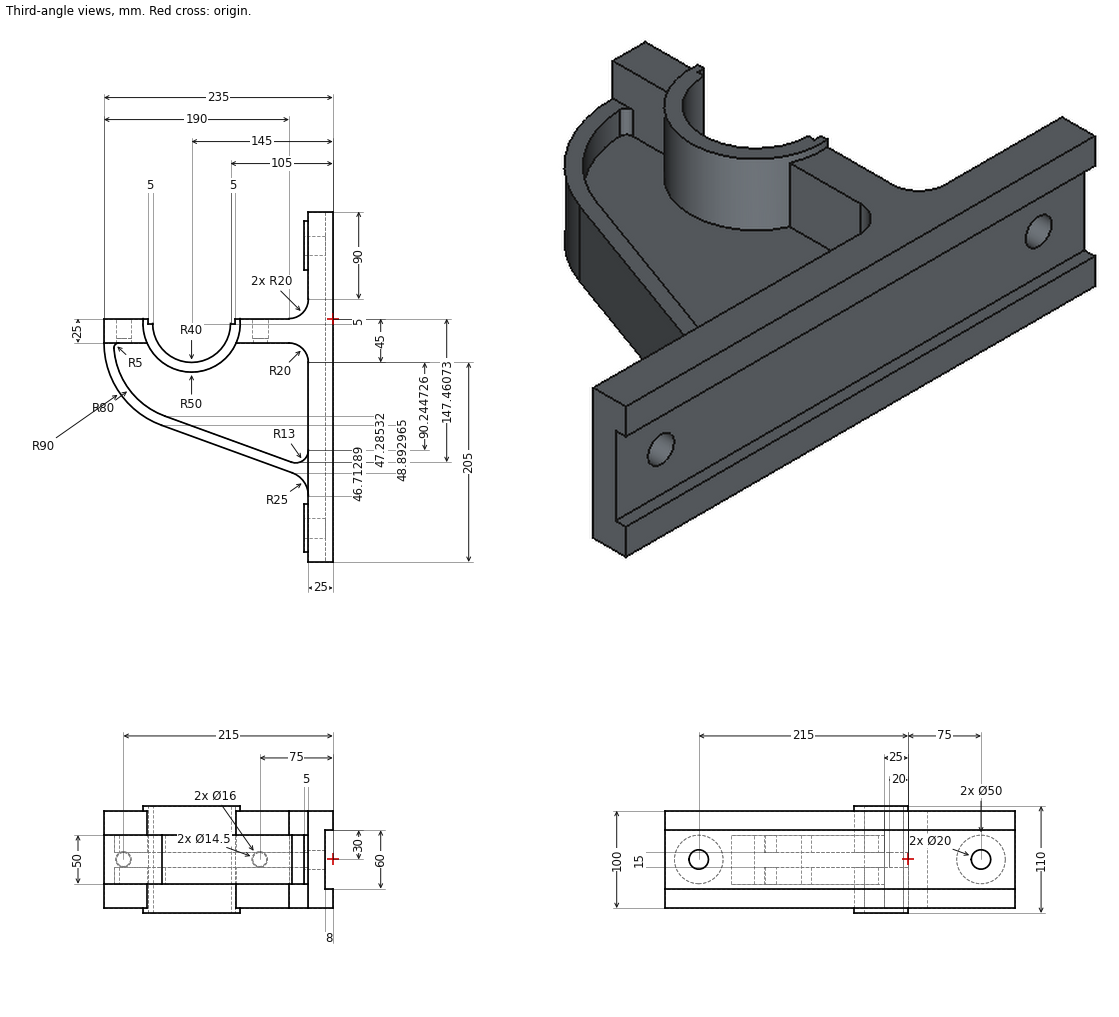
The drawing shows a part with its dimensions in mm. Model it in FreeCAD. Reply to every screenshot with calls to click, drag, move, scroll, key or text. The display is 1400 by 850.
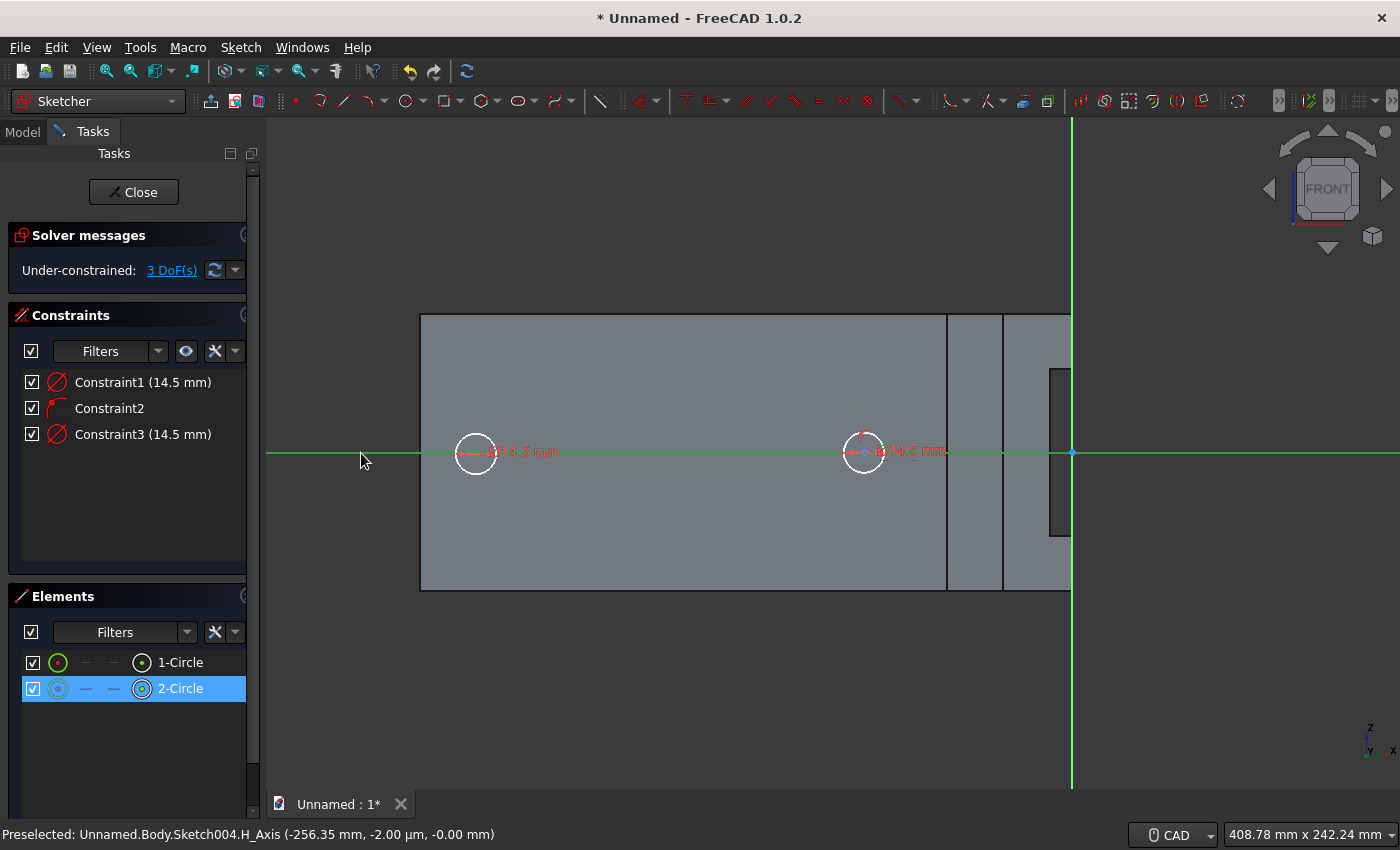
click(686, 102)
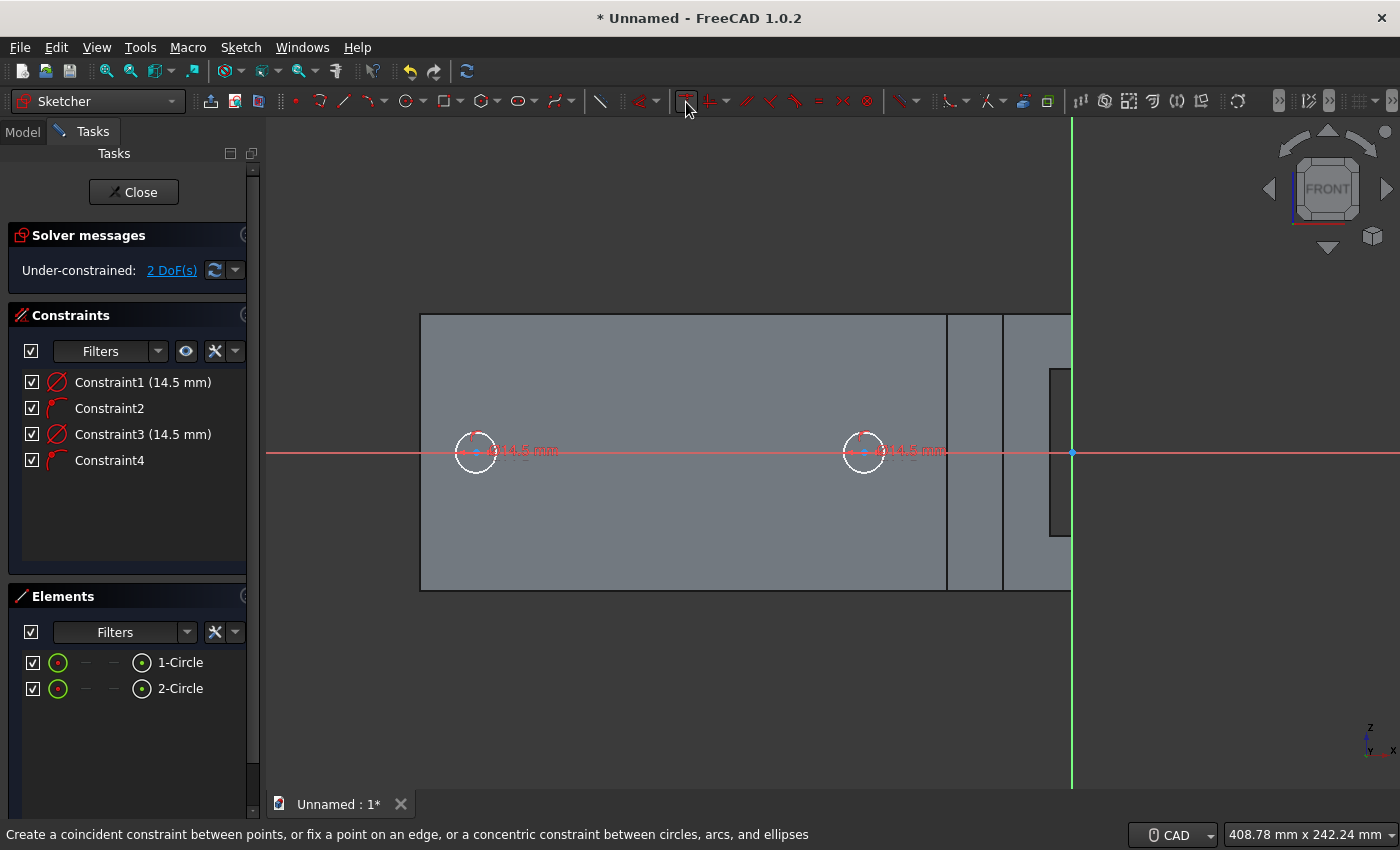
click(640, 102)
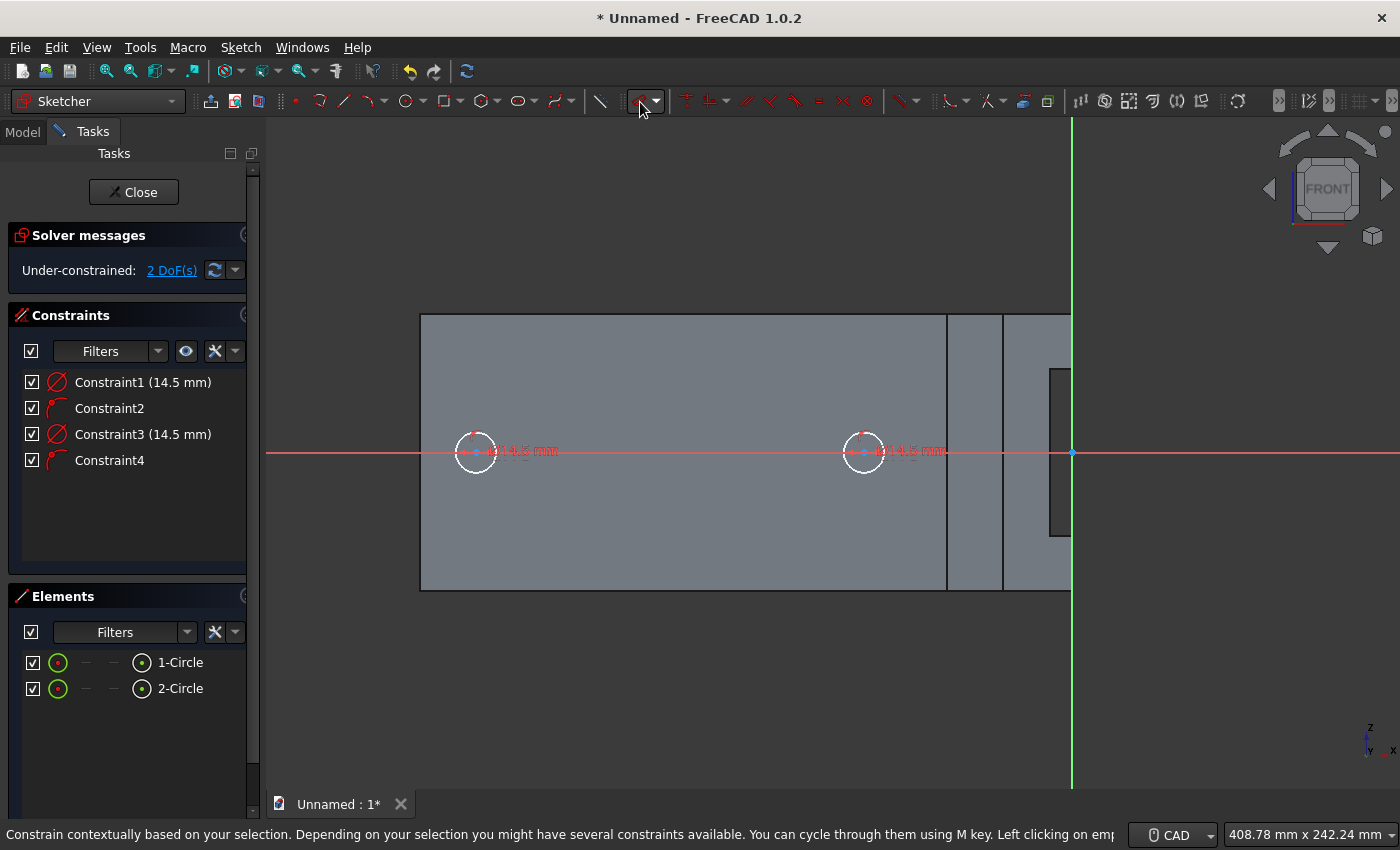
click(864, 453)
click(968, 487)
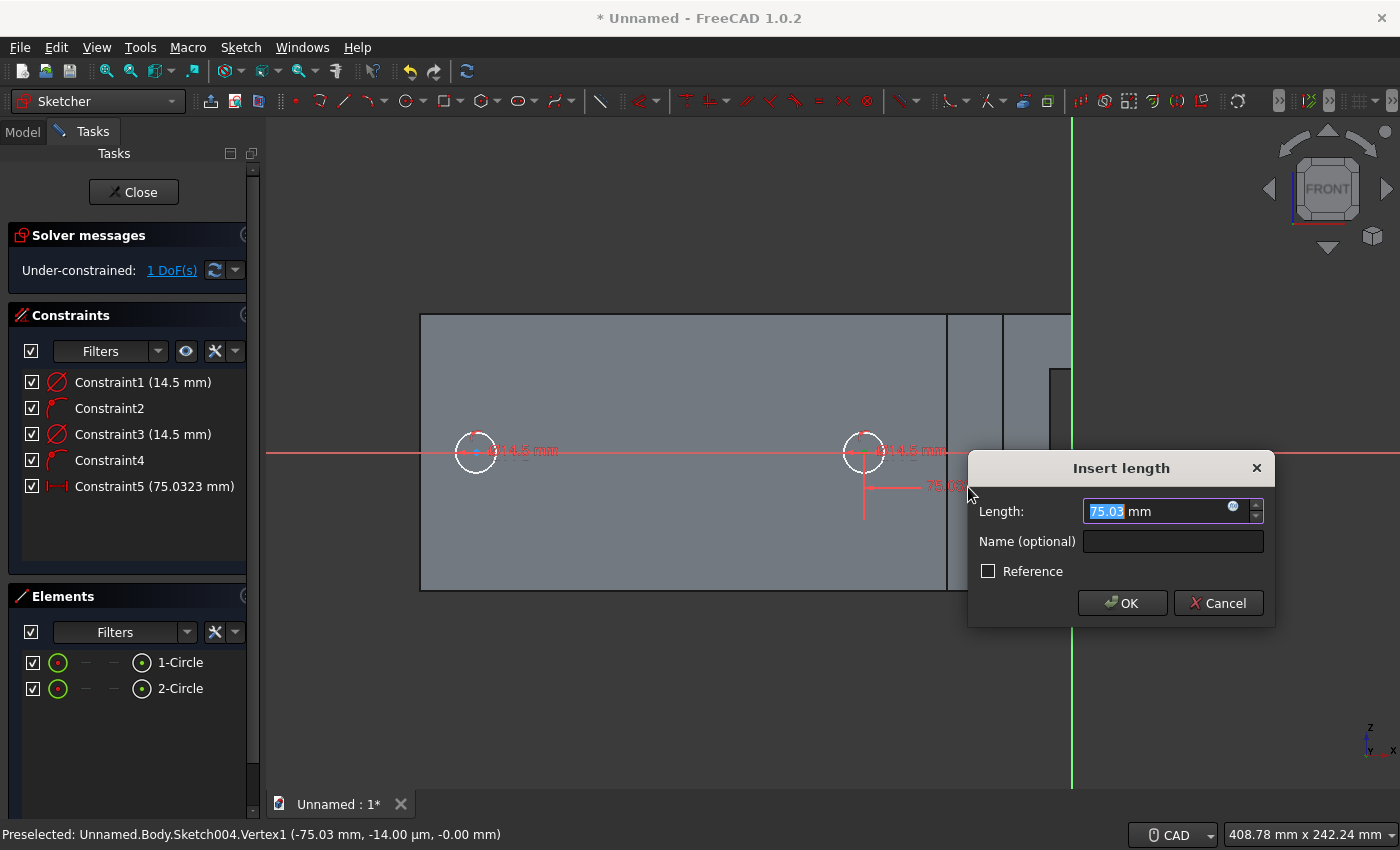
text(75)
key(Return)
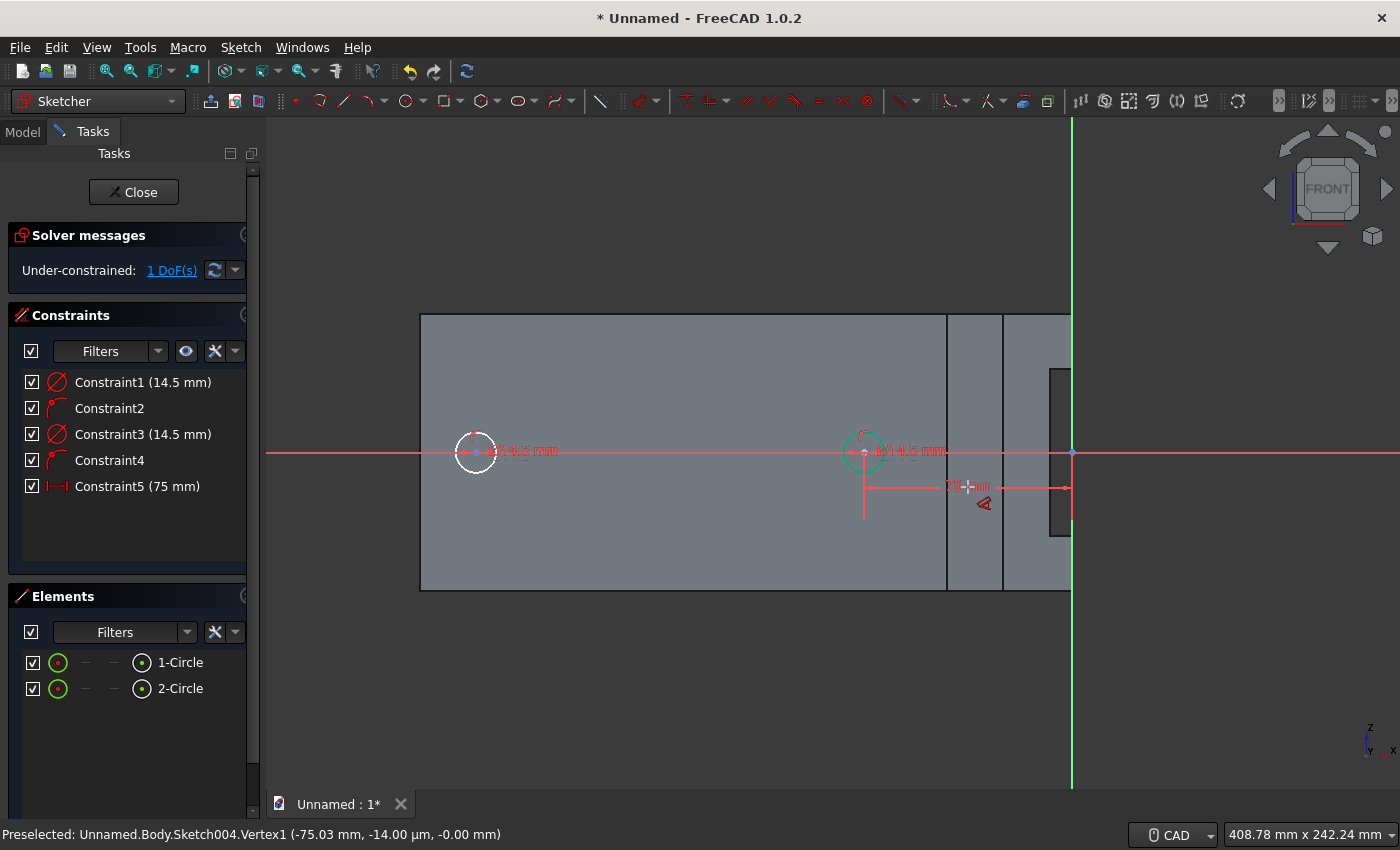
click(476, 453)
click(774, 487)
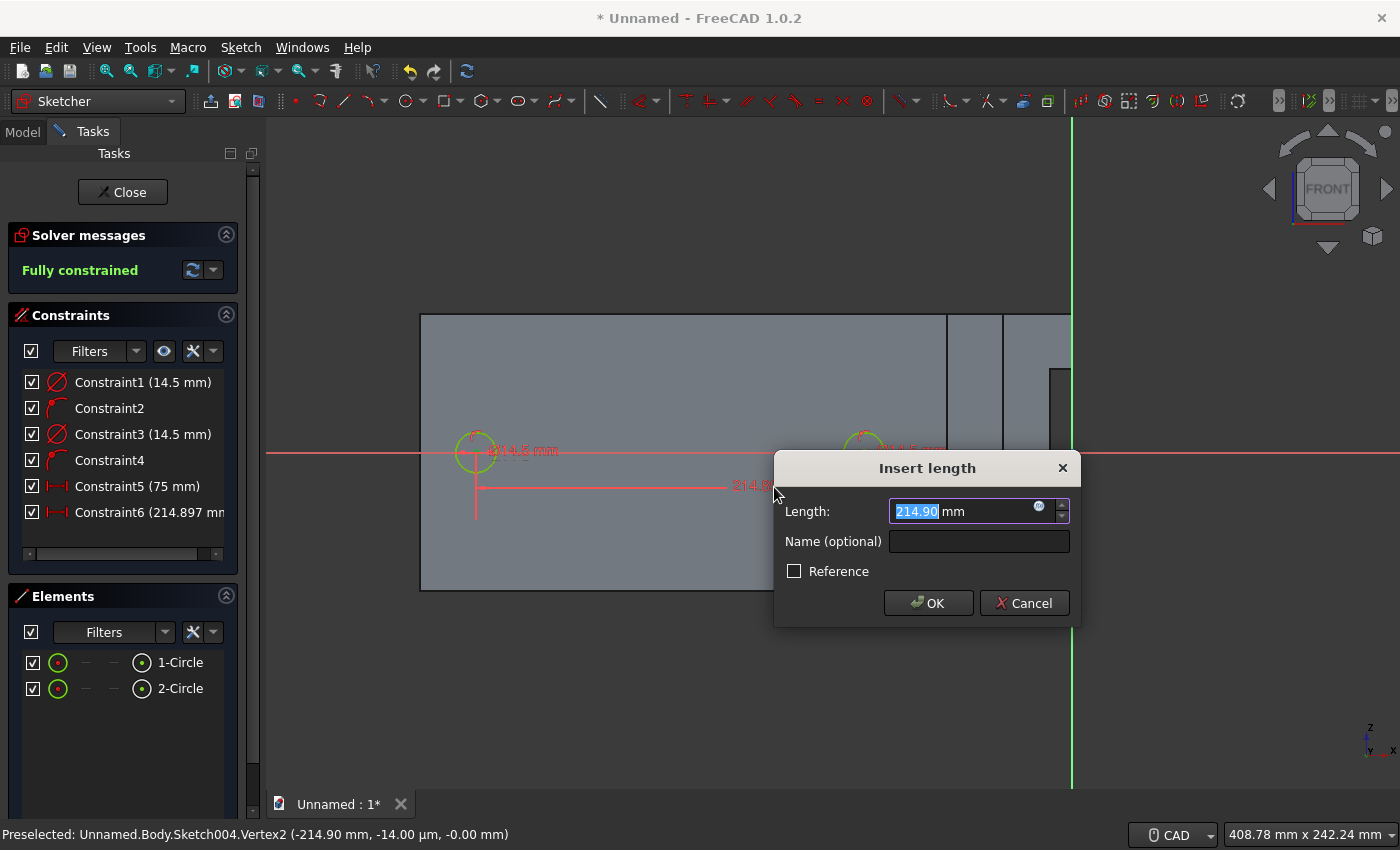
text(215)
key(Return)
key(Escape)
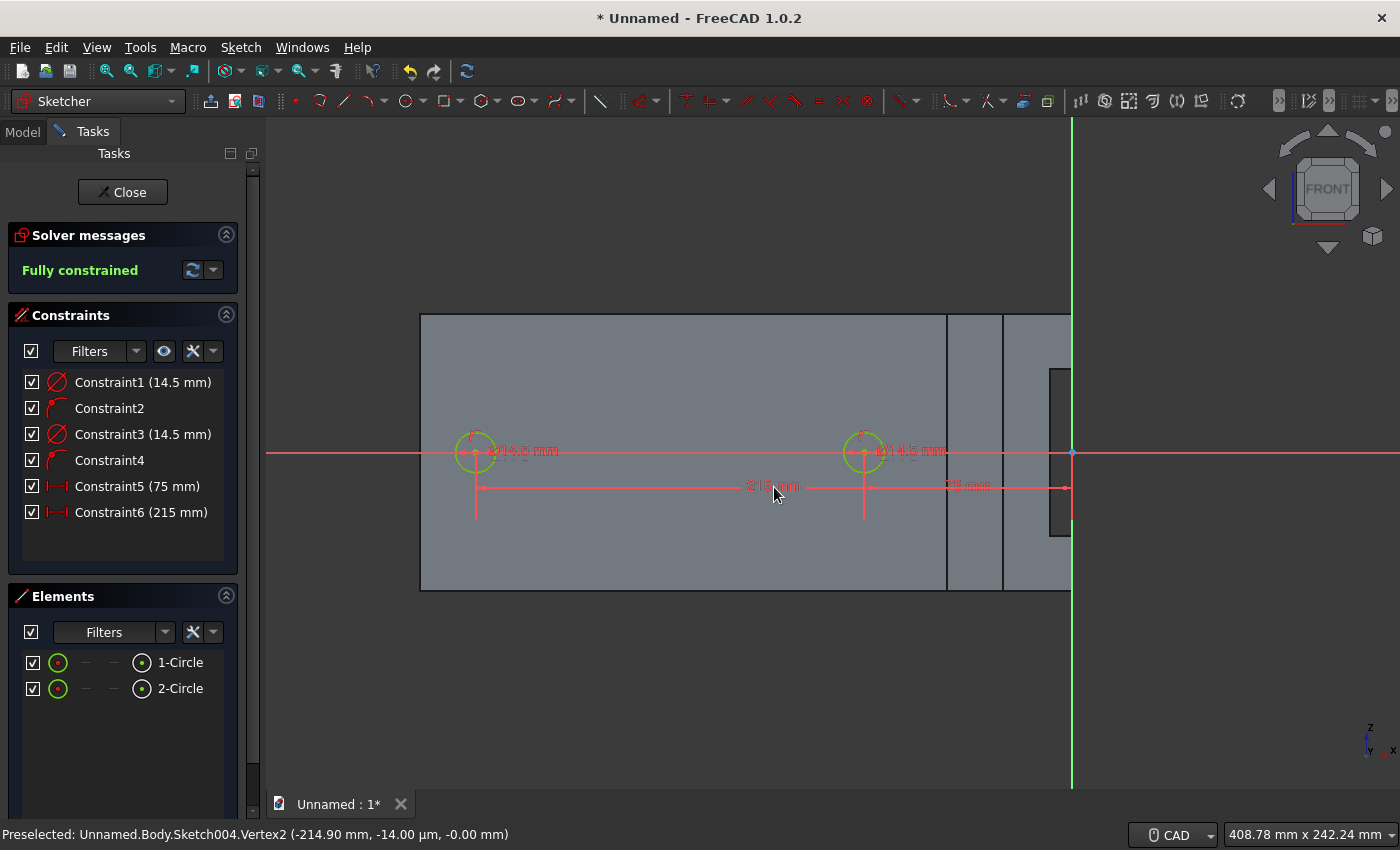
click(123, 192)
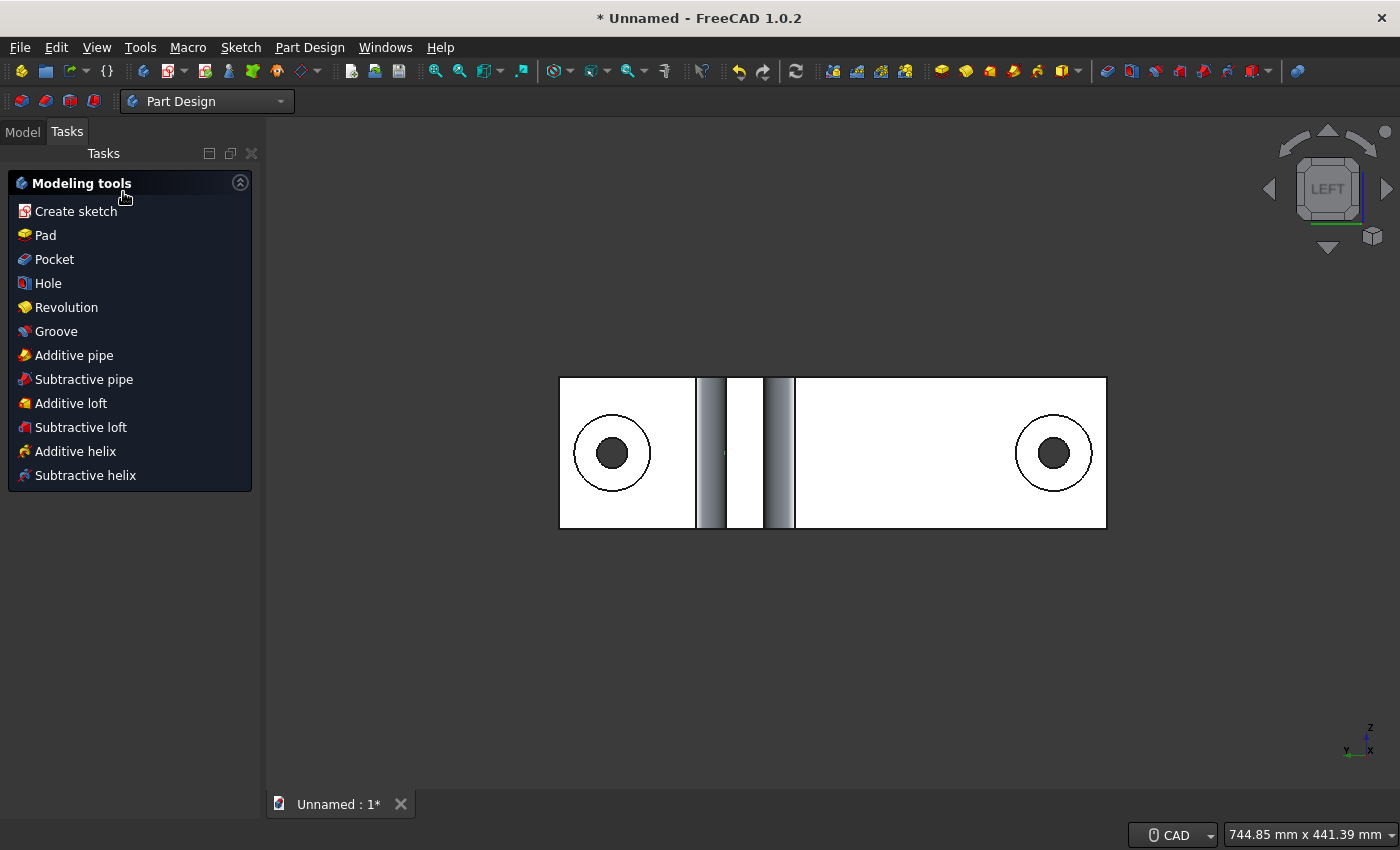
click(1108, 72)